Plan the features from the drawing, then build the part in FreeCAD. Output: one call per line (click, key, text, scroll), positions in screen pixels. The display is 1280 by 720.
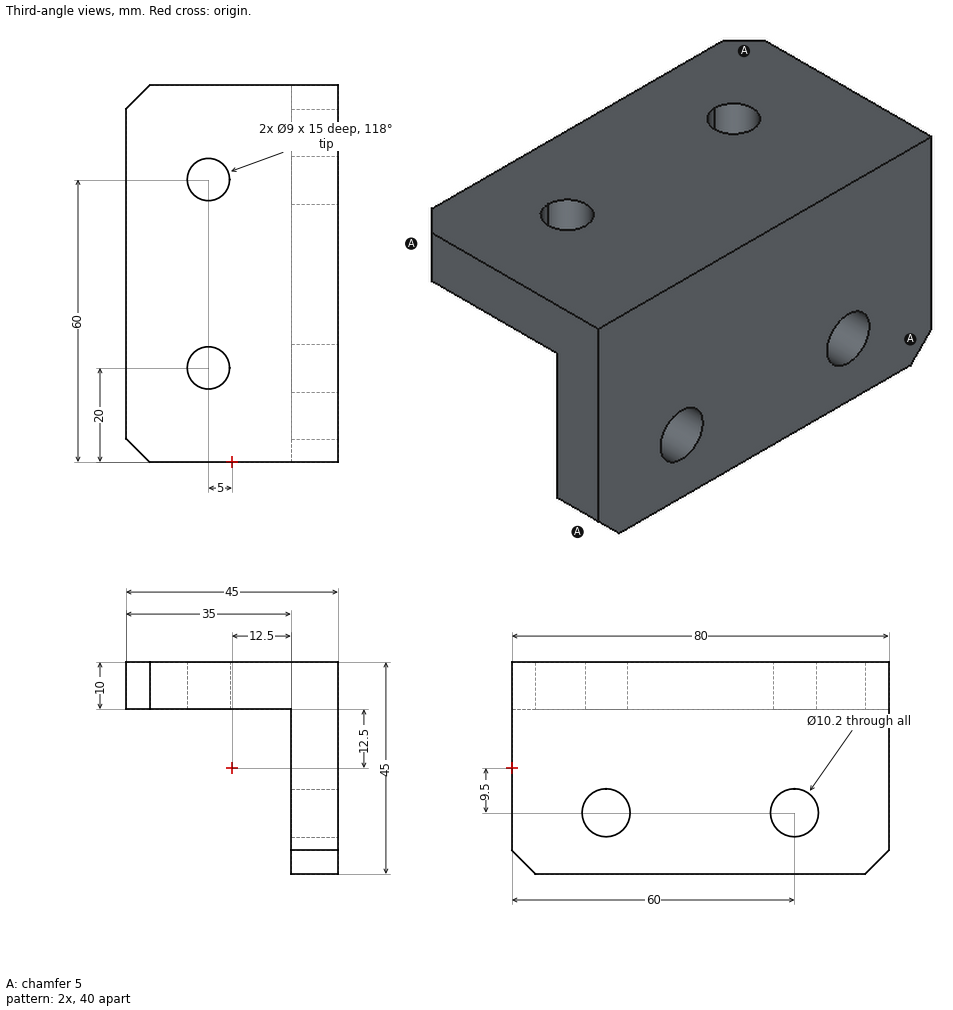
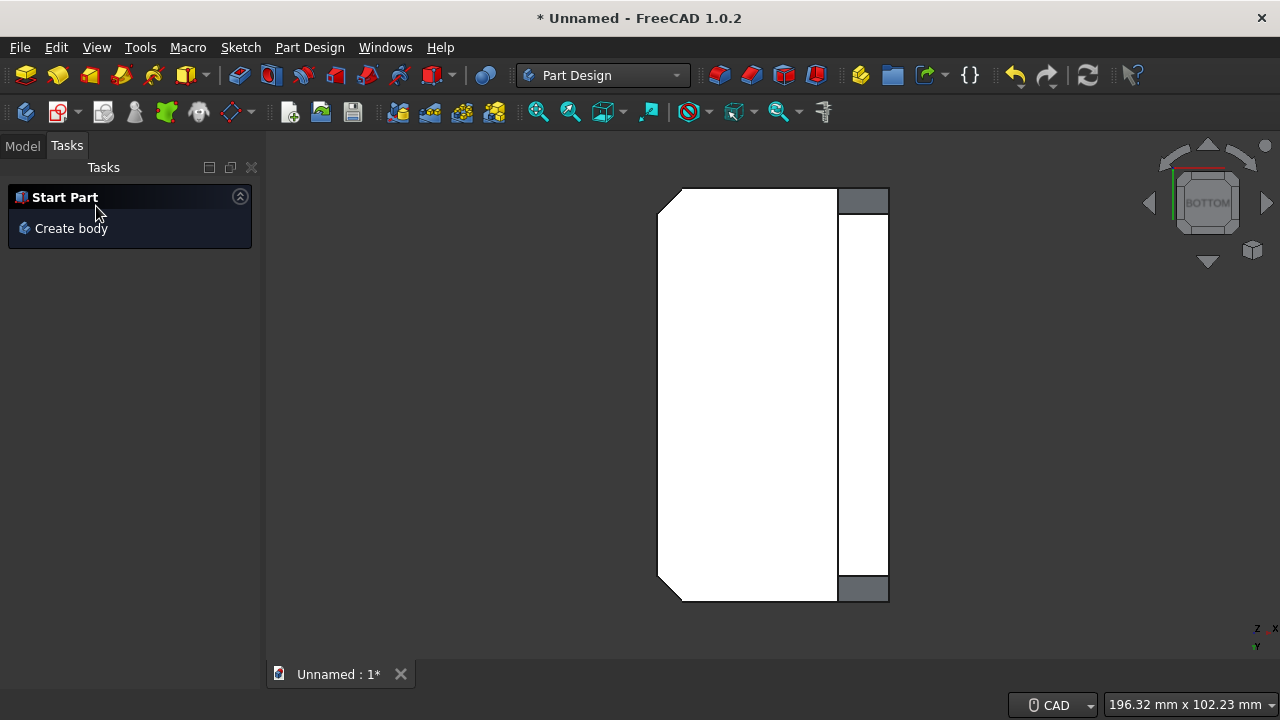
click(747, 453)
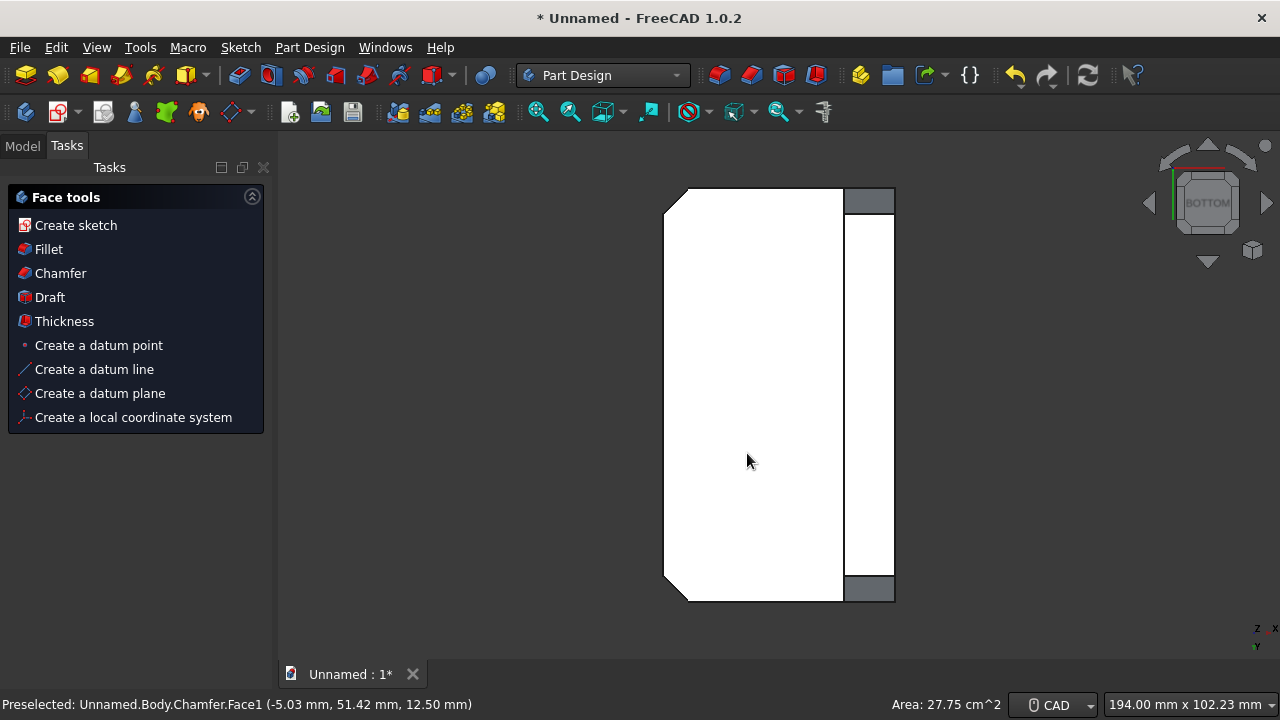
click(58, 112)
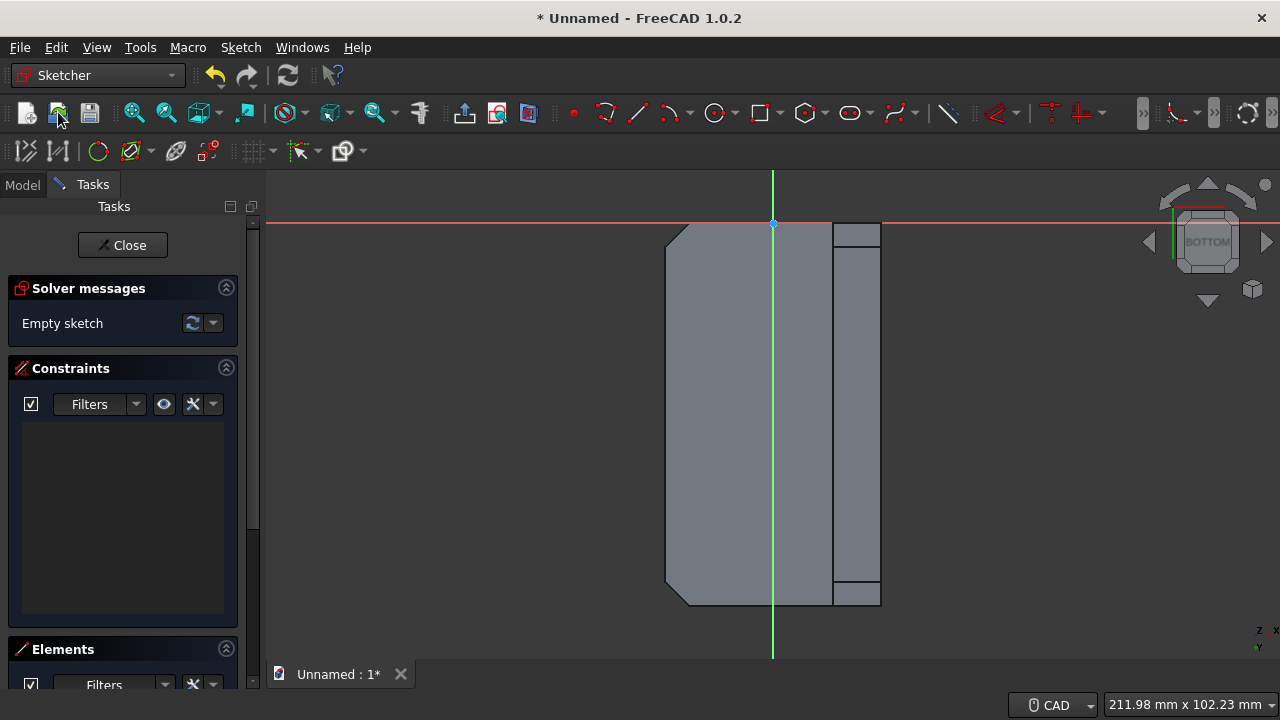
key(q)
key(s)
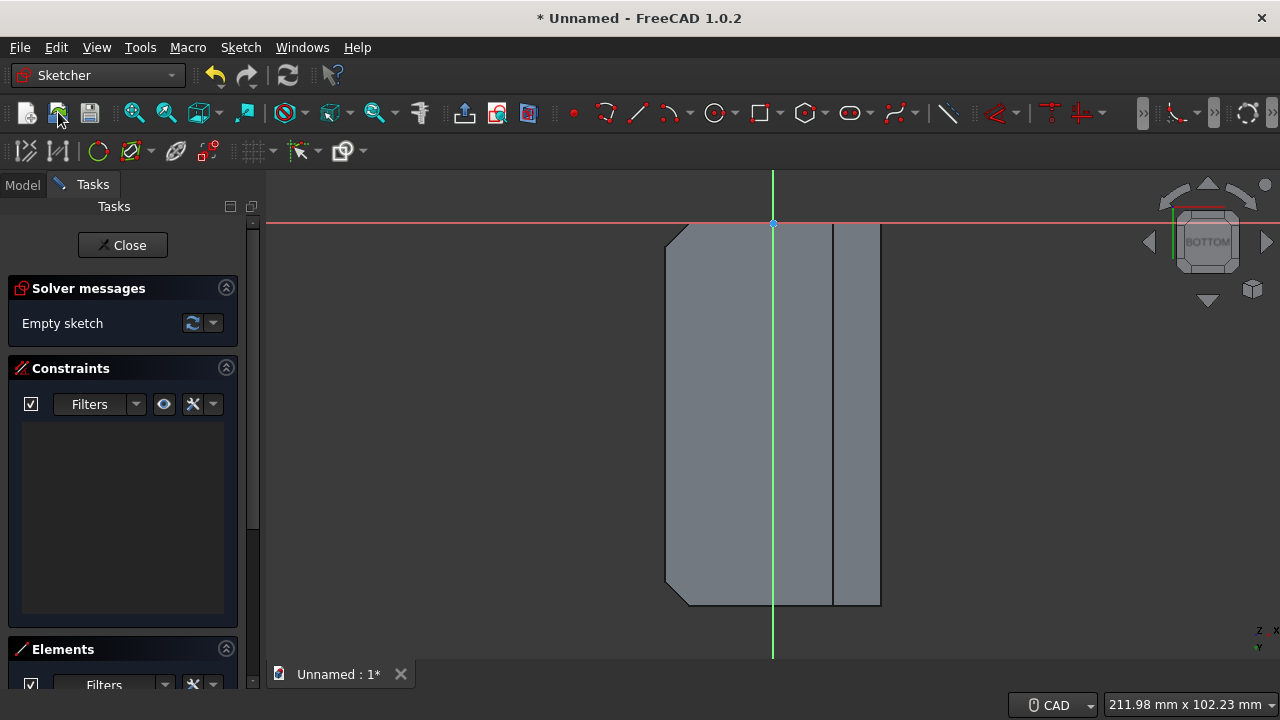
key(g)
key(c)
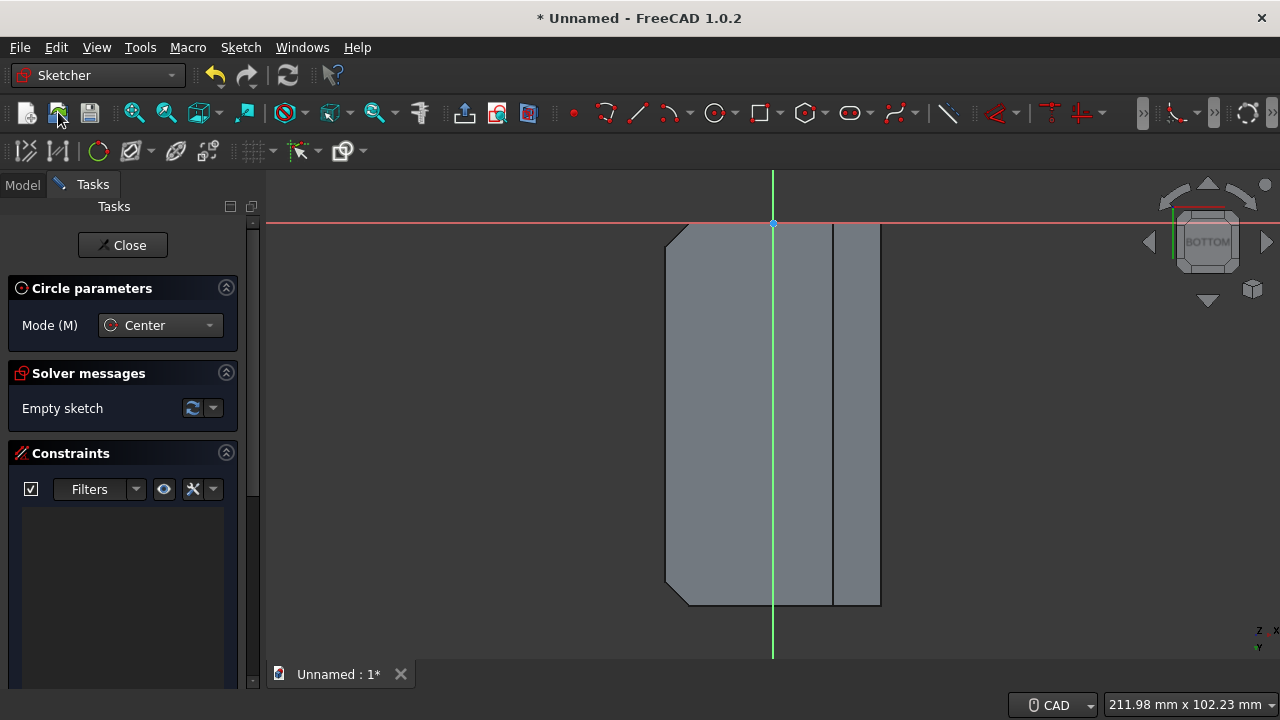
click(749, 510)
move(734, 495)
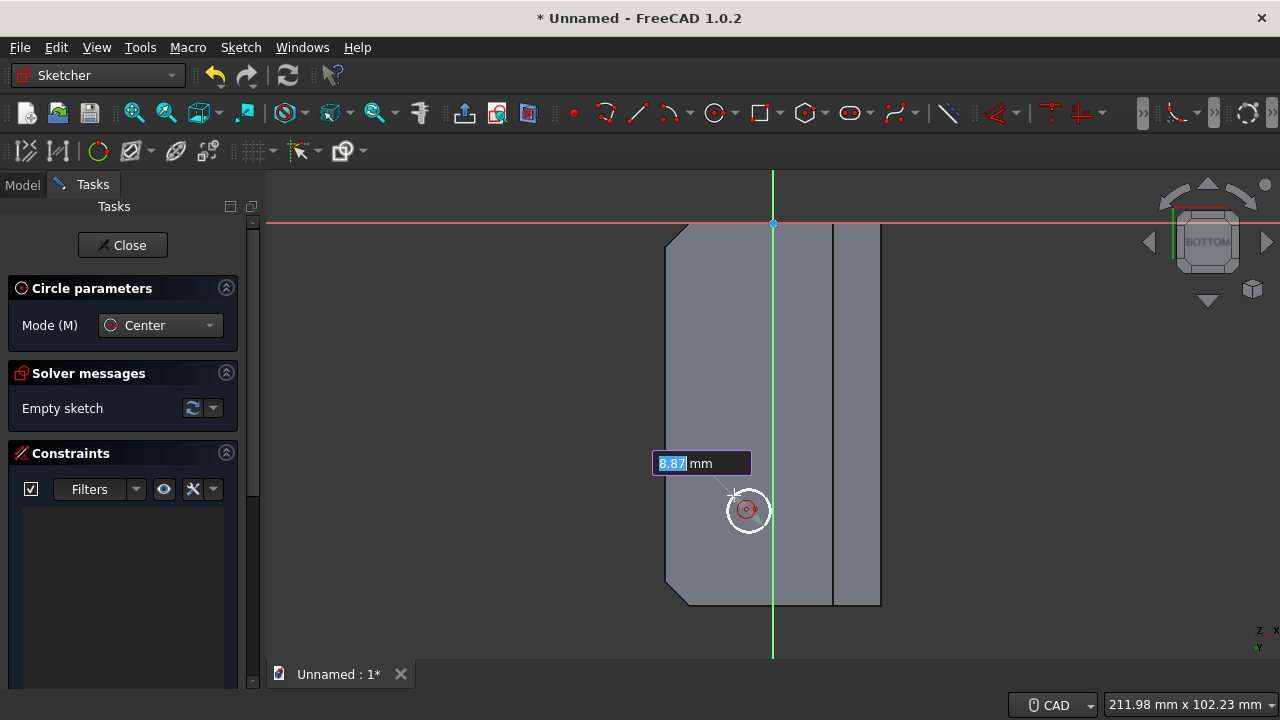
text(9)
key(Return)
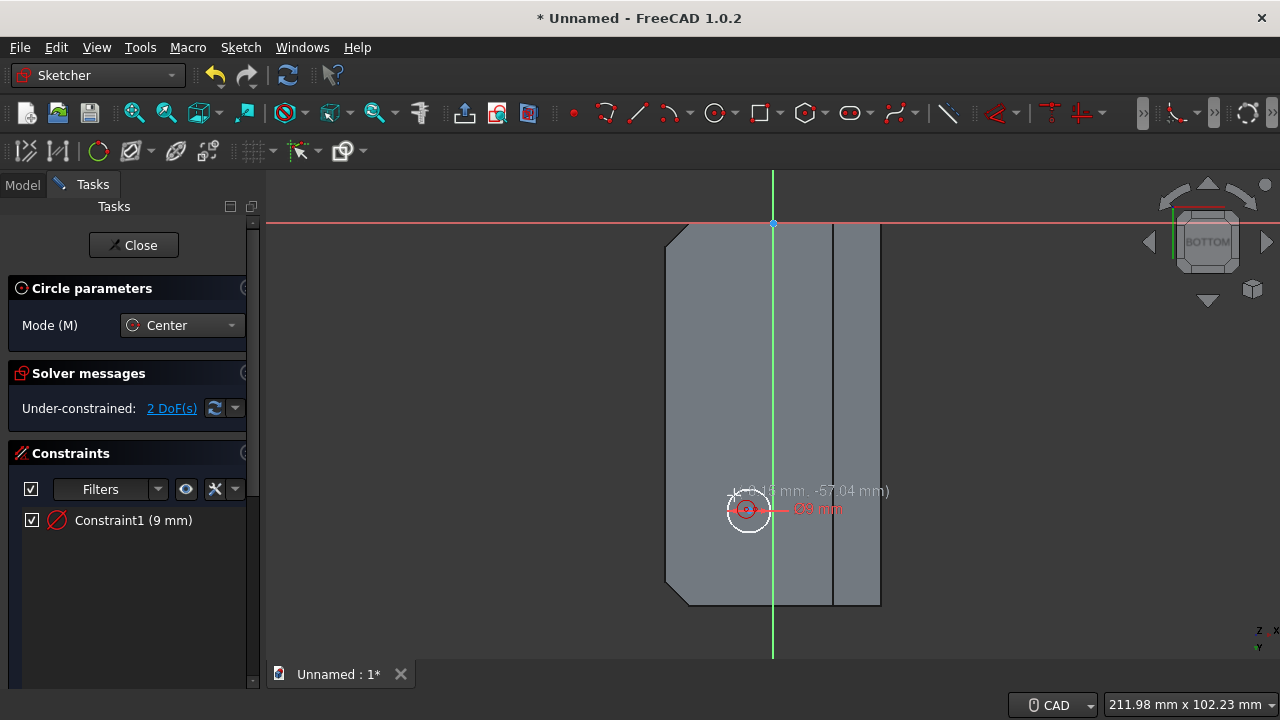
click(749, 319)
move(734, 304)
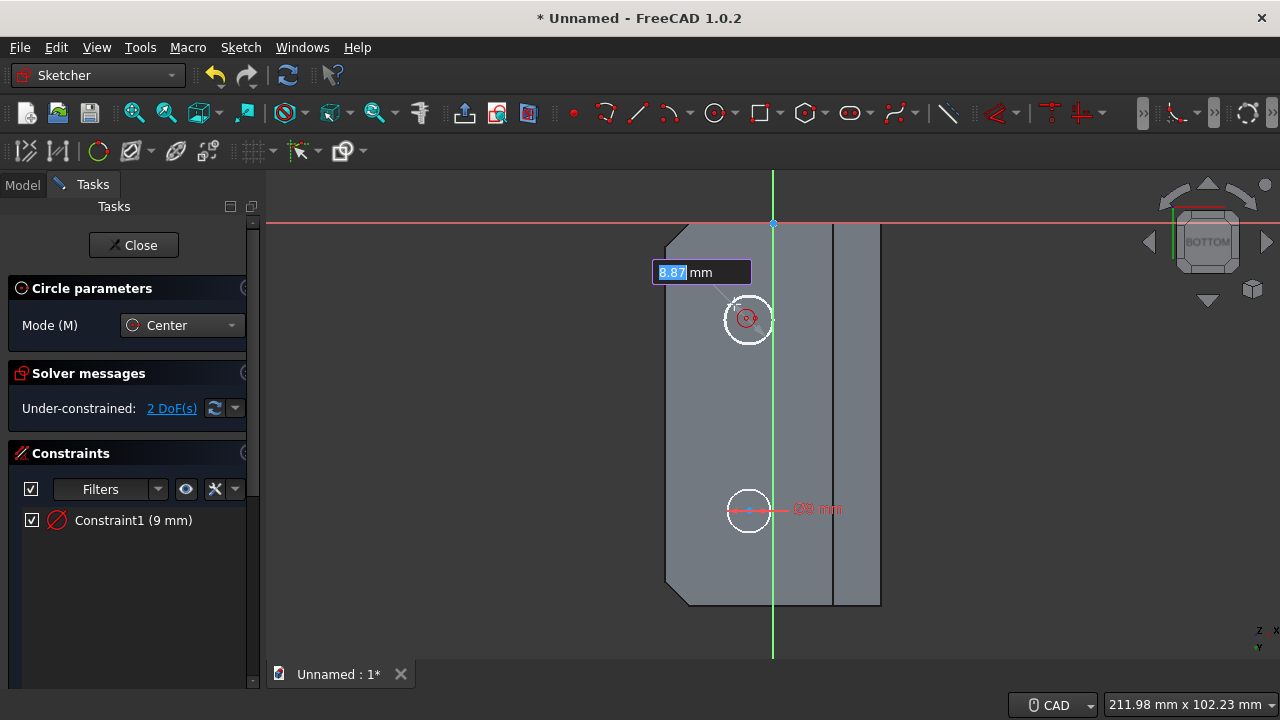
text(9)
key(Return)
key(Escape)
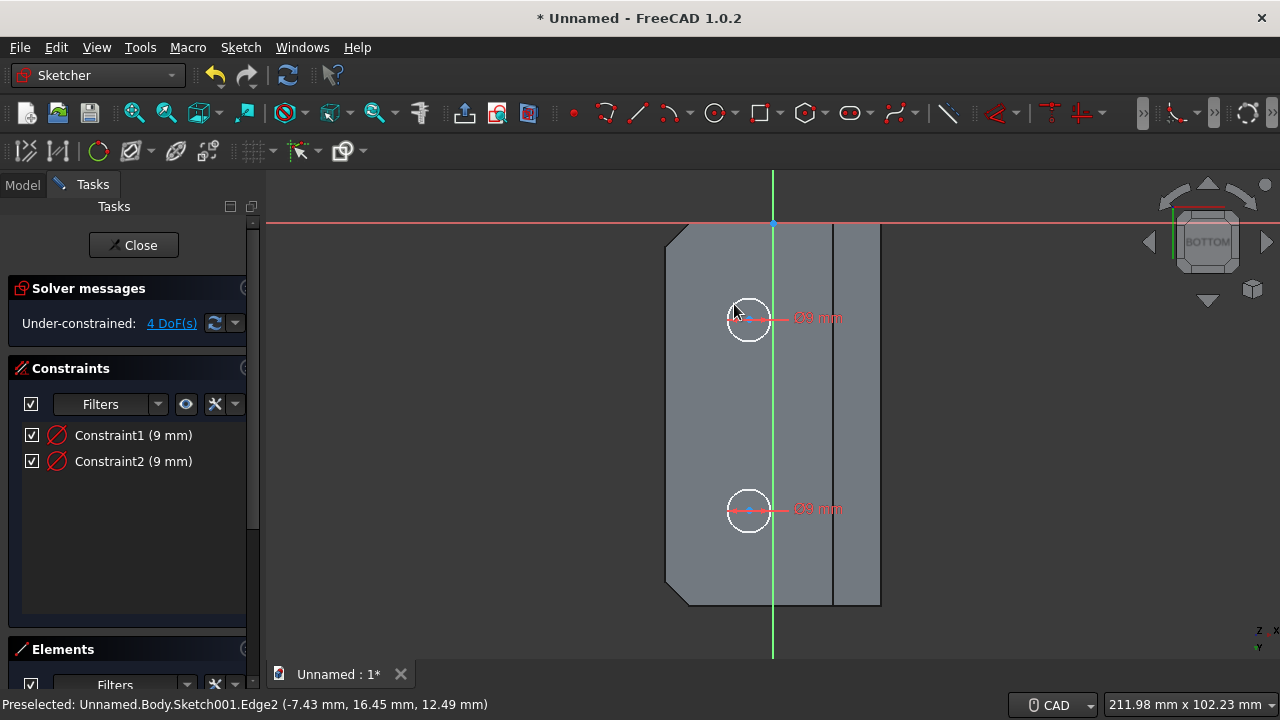
key(d)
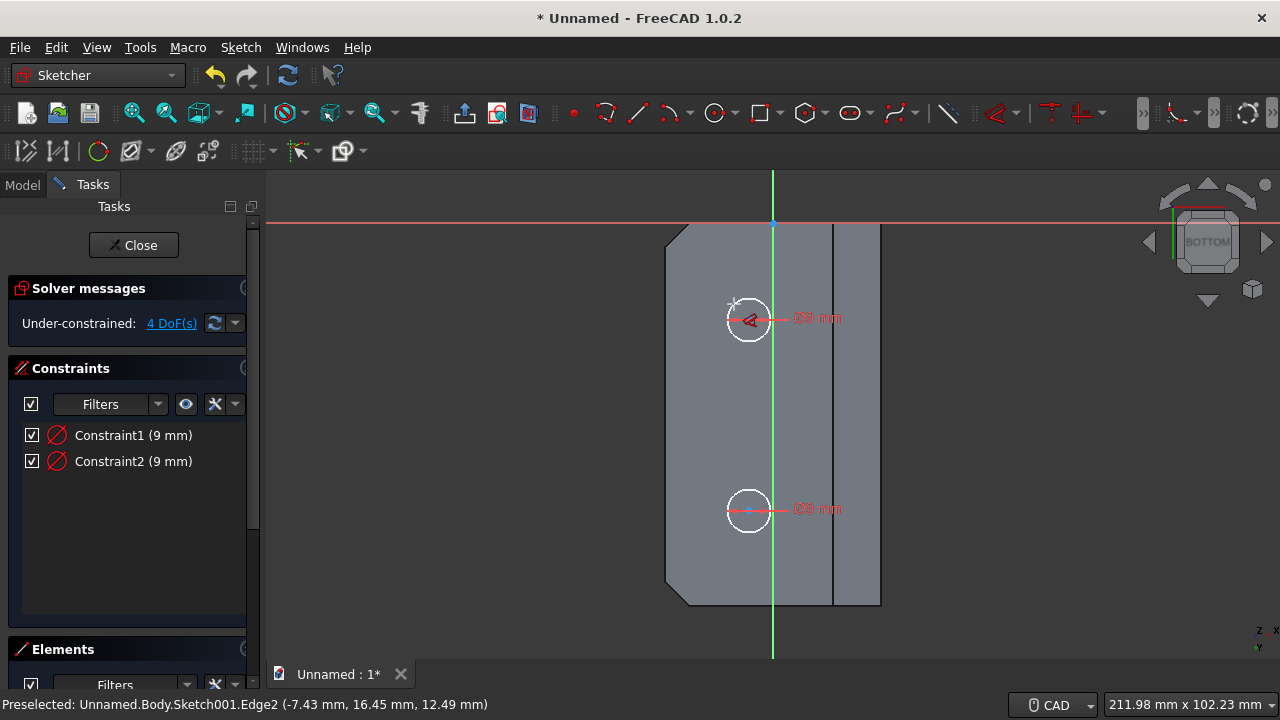
scroll(749, 511, up, 3)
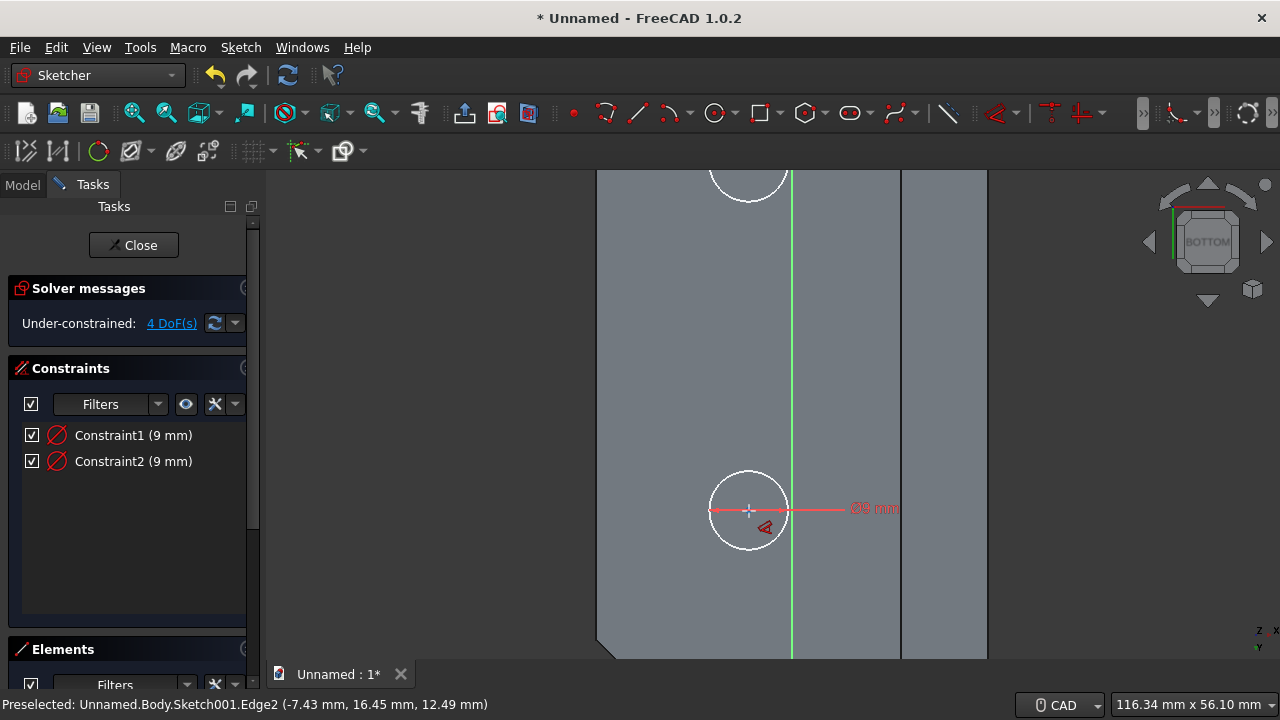
click(749, 510)
click(770, 568)